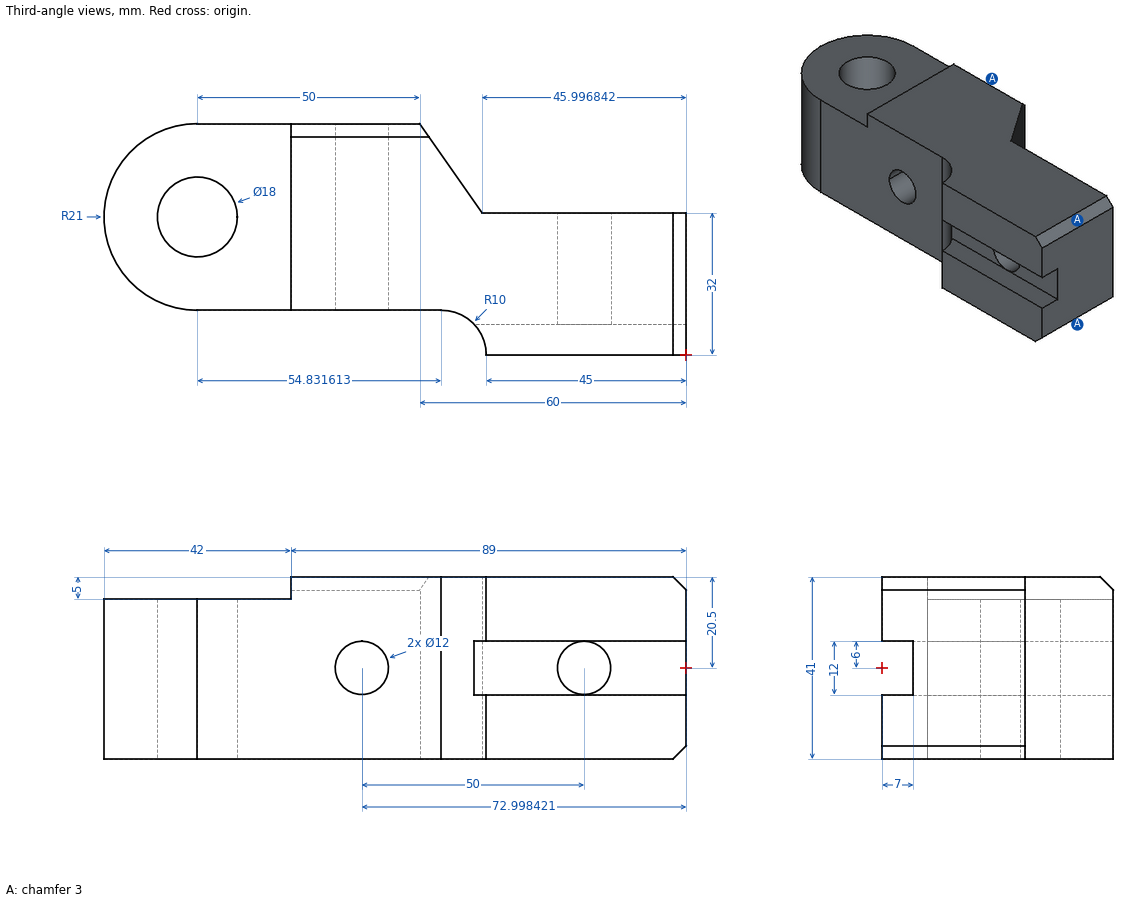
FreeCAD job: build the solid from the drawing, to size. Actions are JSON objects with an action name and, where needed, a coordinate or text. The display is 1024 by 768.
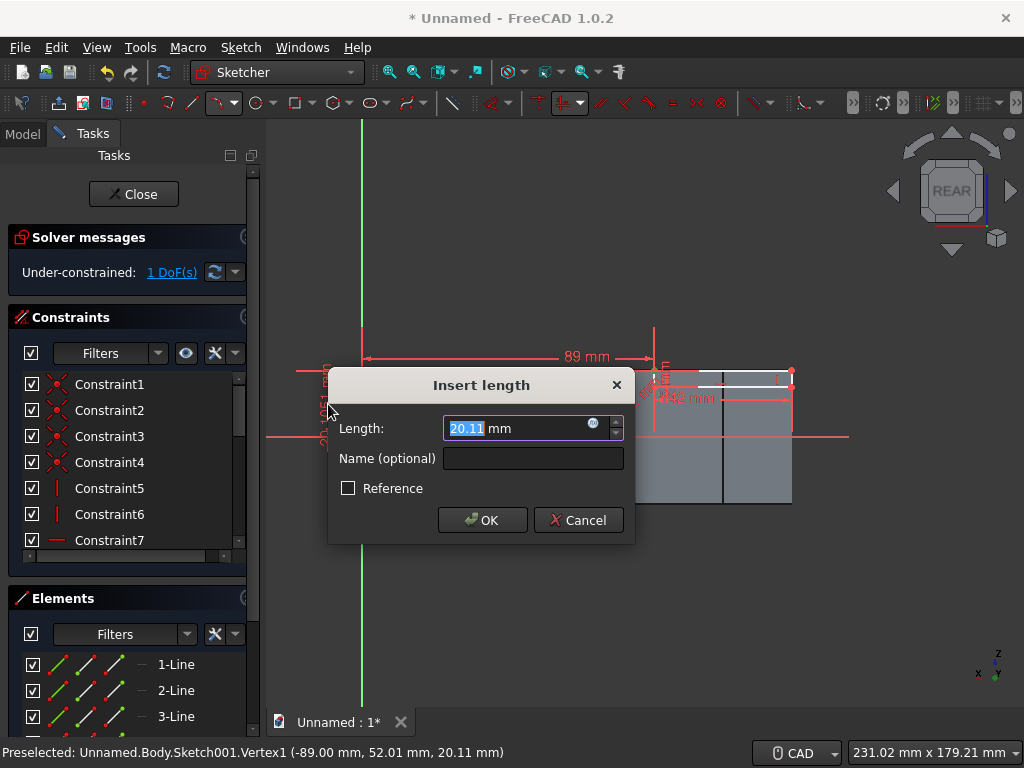
{"action": "type", "text": "20.5"}
{"action": "key", "text": "Return"}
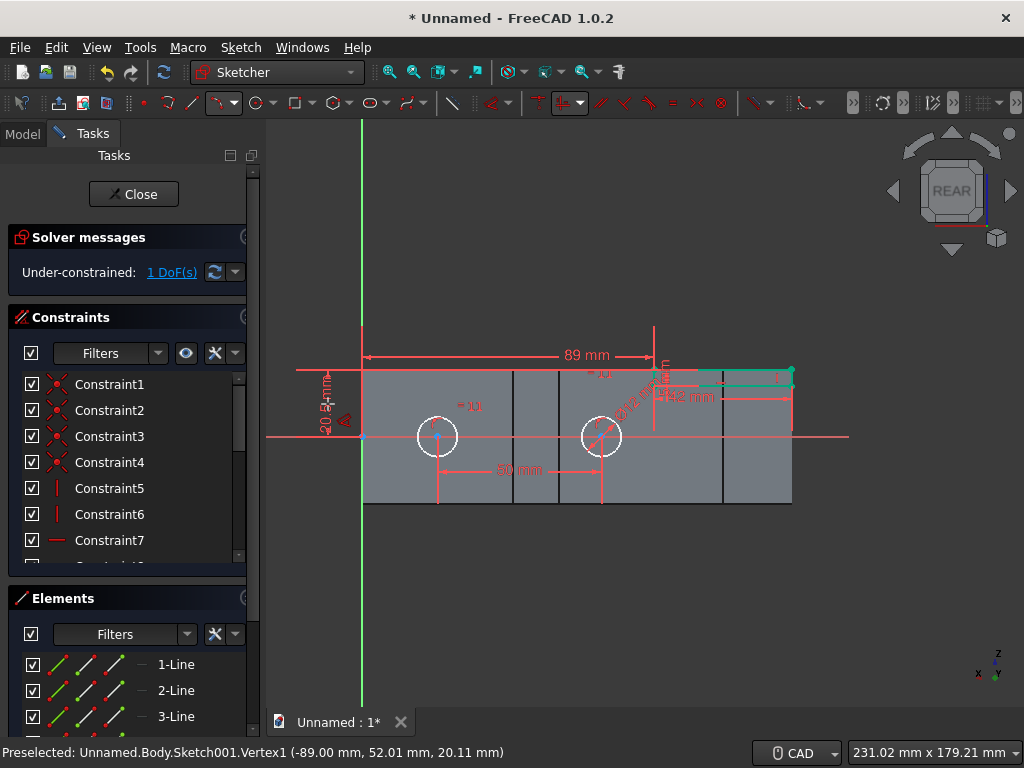
{"action": "left_click", "coordinate": [602, 437]}
{"action": "left_click", "coordinate": [427, 471]}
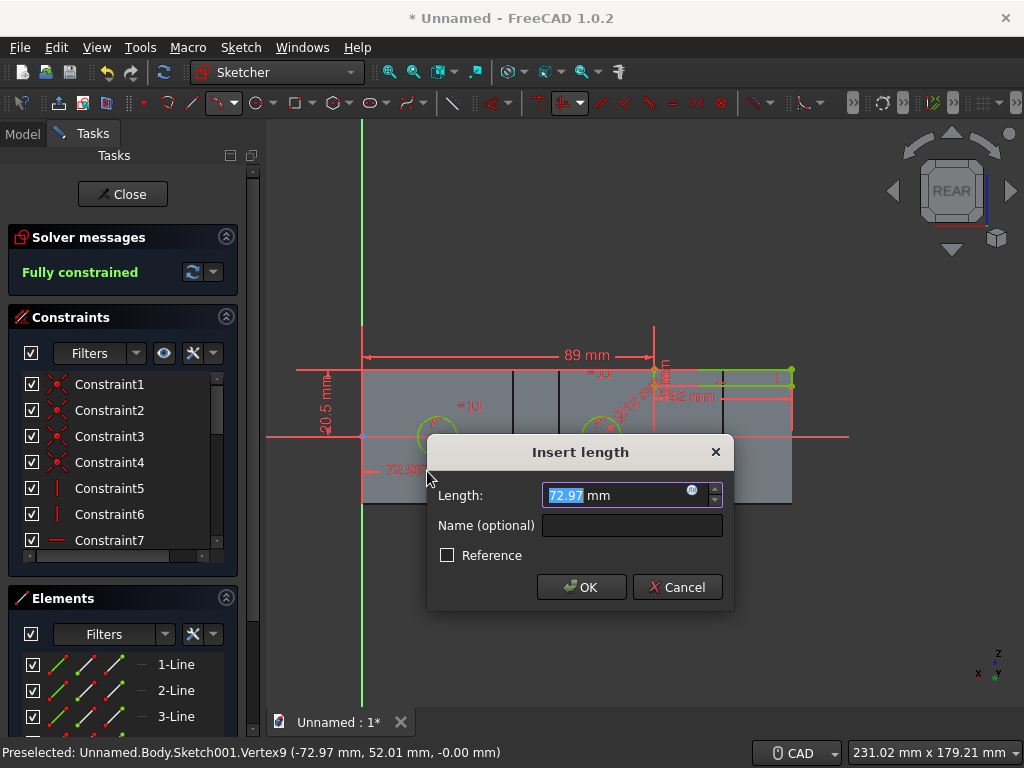
{"action": "type", "text": "72.998421"}
{"action": "key", "text": "Return"}
{"action": "key", "text": "Escape"}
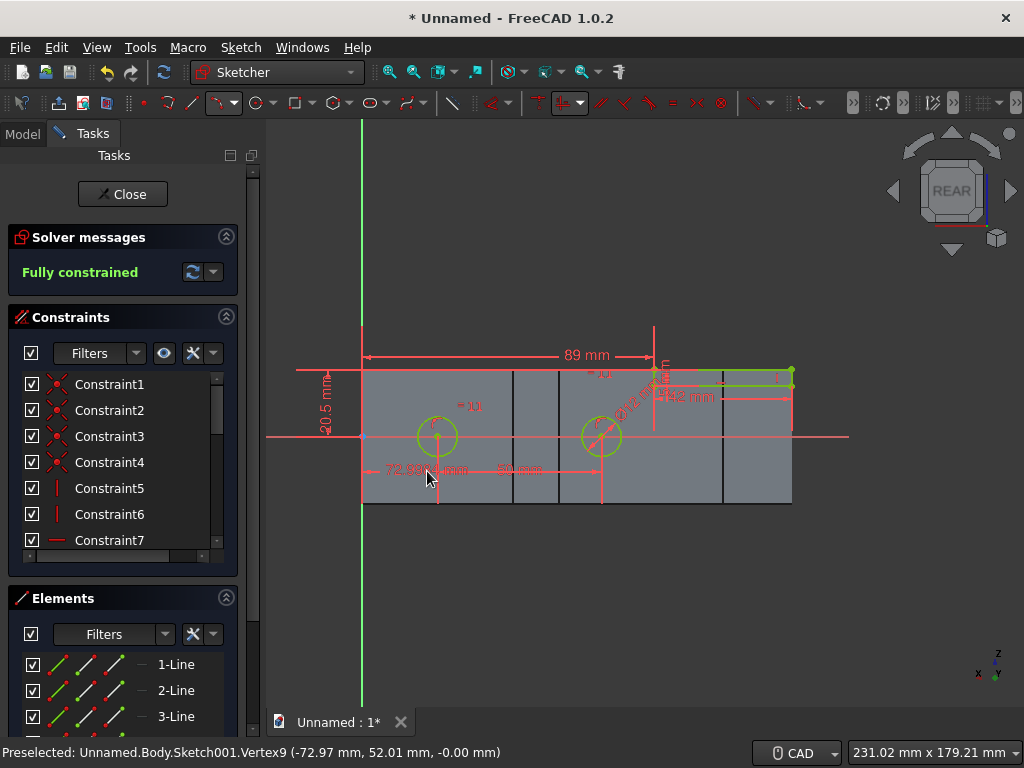
{"action": "left_click", "coordinate": [123, 194]}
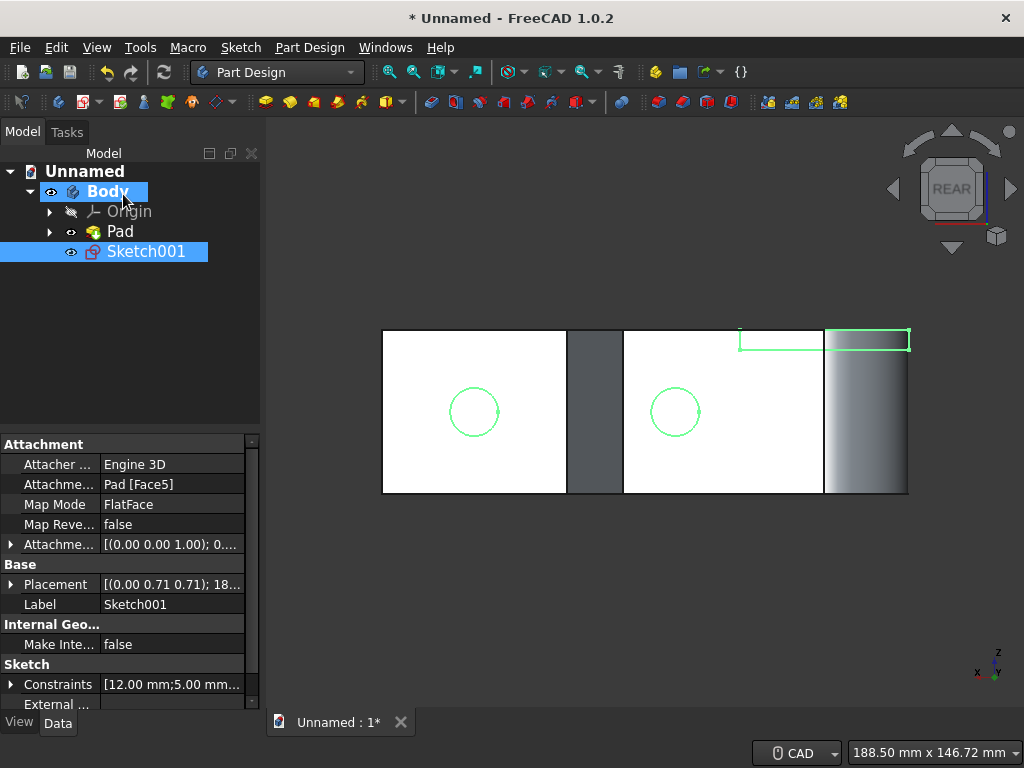
{"action": "left_click", "coordinate": [432, 102]}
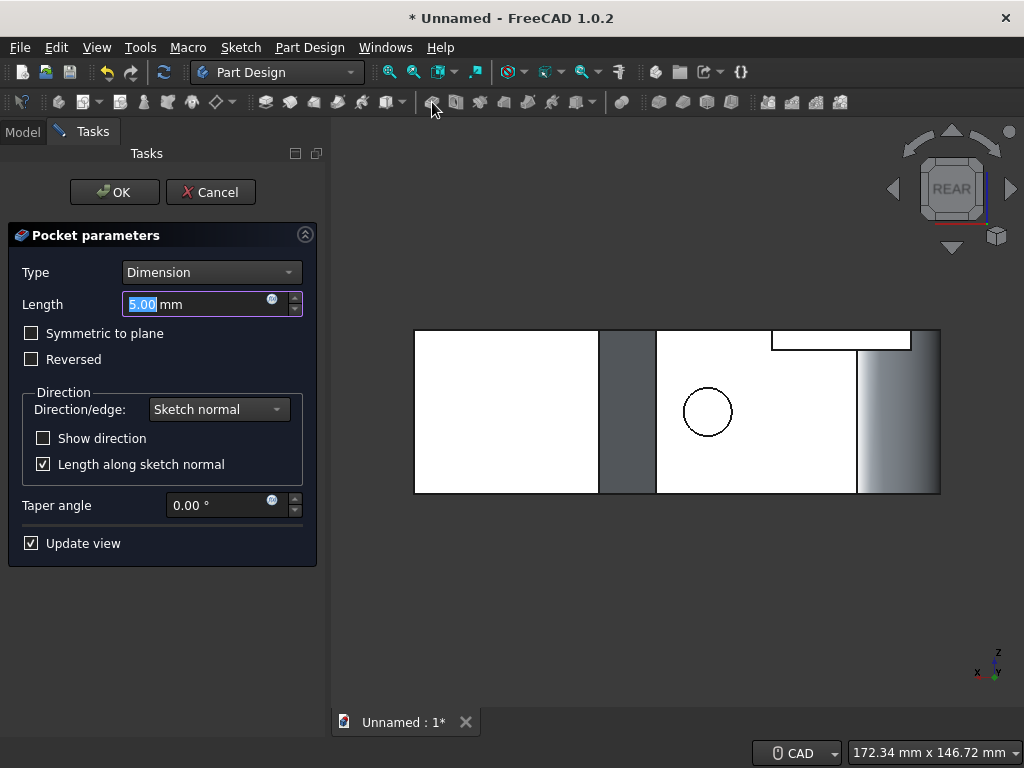
{"action": "left_click", "coordinate": [212, 272]}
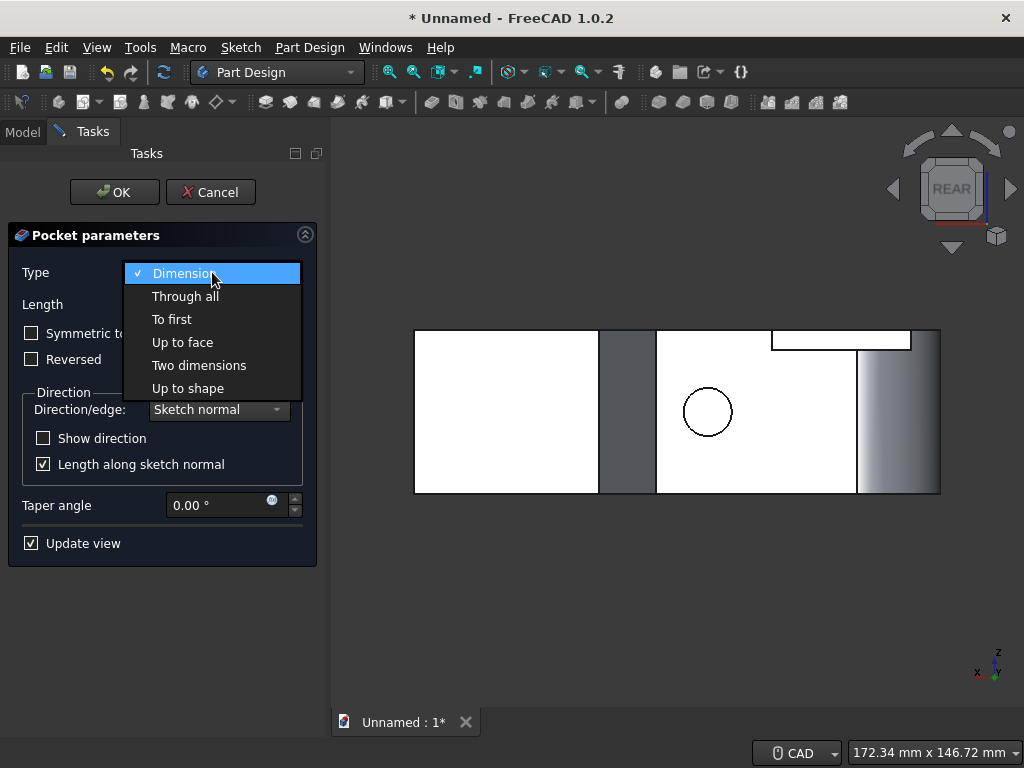
{"action": "left_click", "coordinate": [212, 296]}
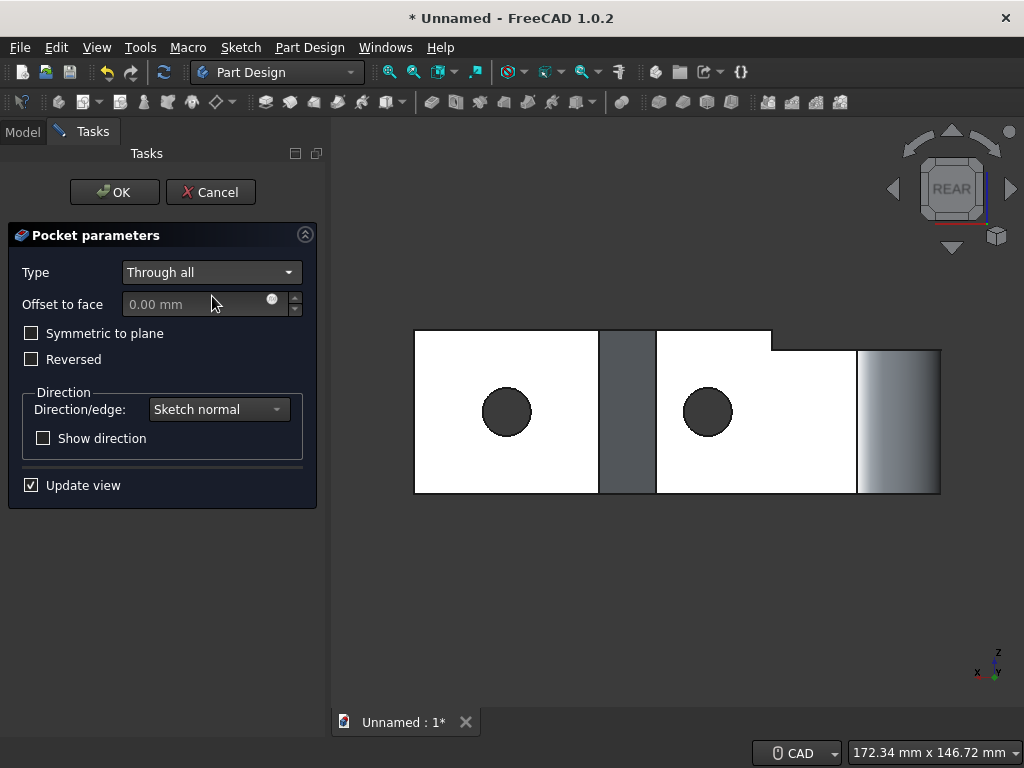
{"action": "left_click", "coordinate": [115, 192]}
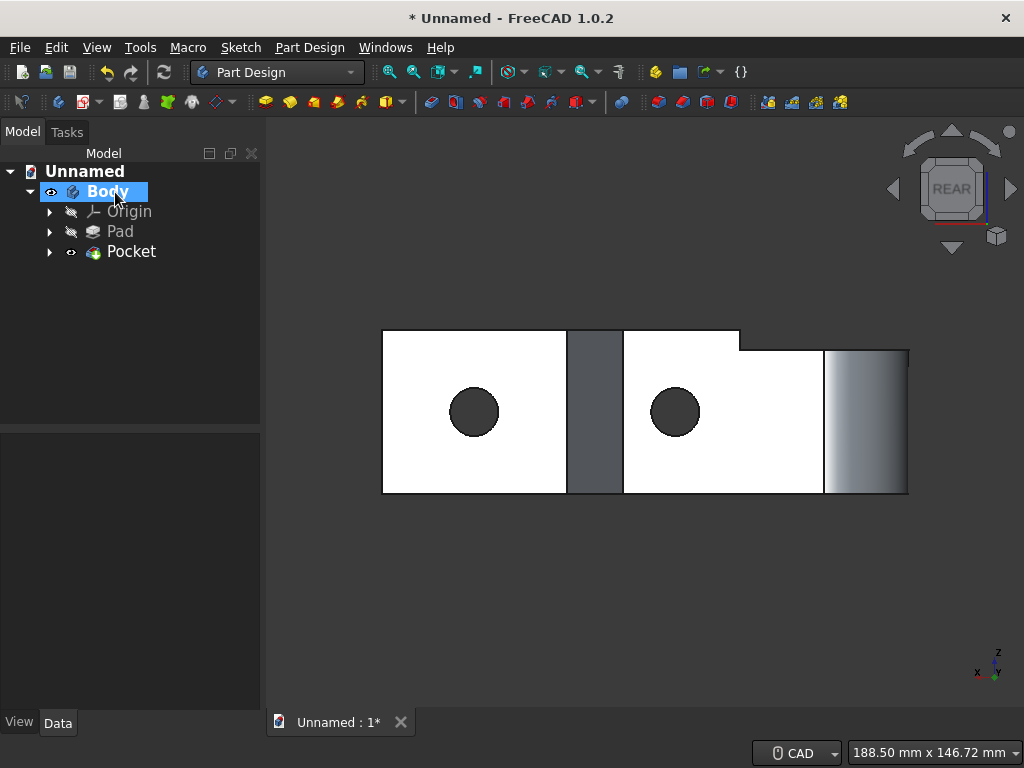
{"action": "left_click", "coordinate": [84, 102]}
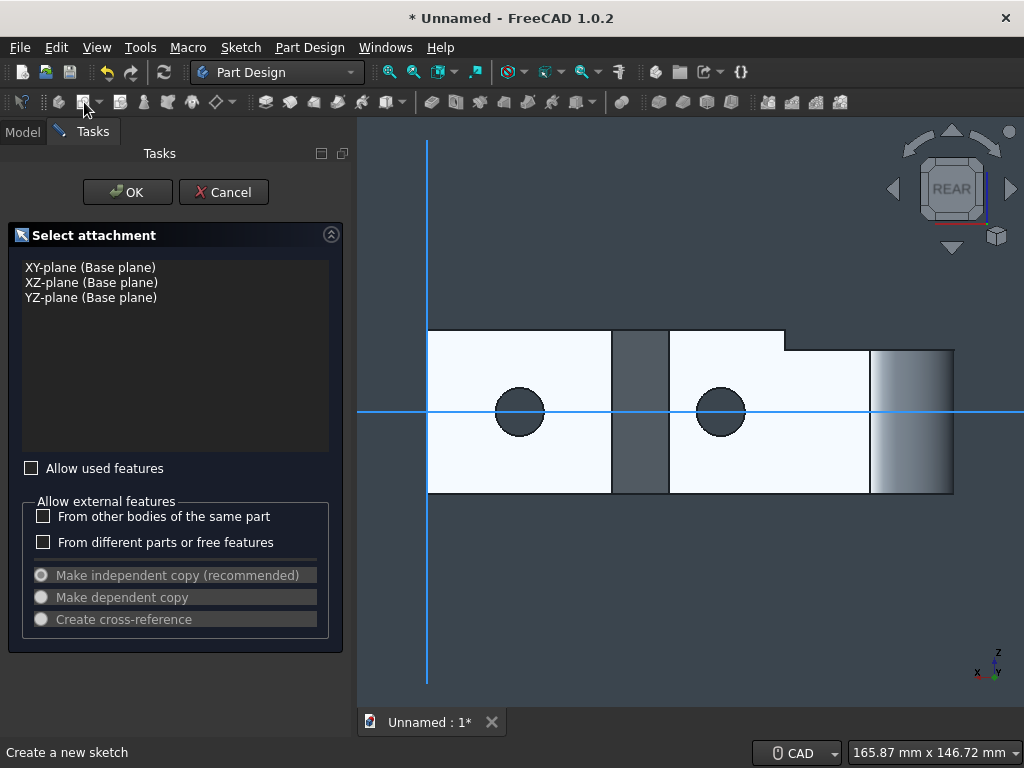
{"action": "left_click", "coordinate": [82, 298]}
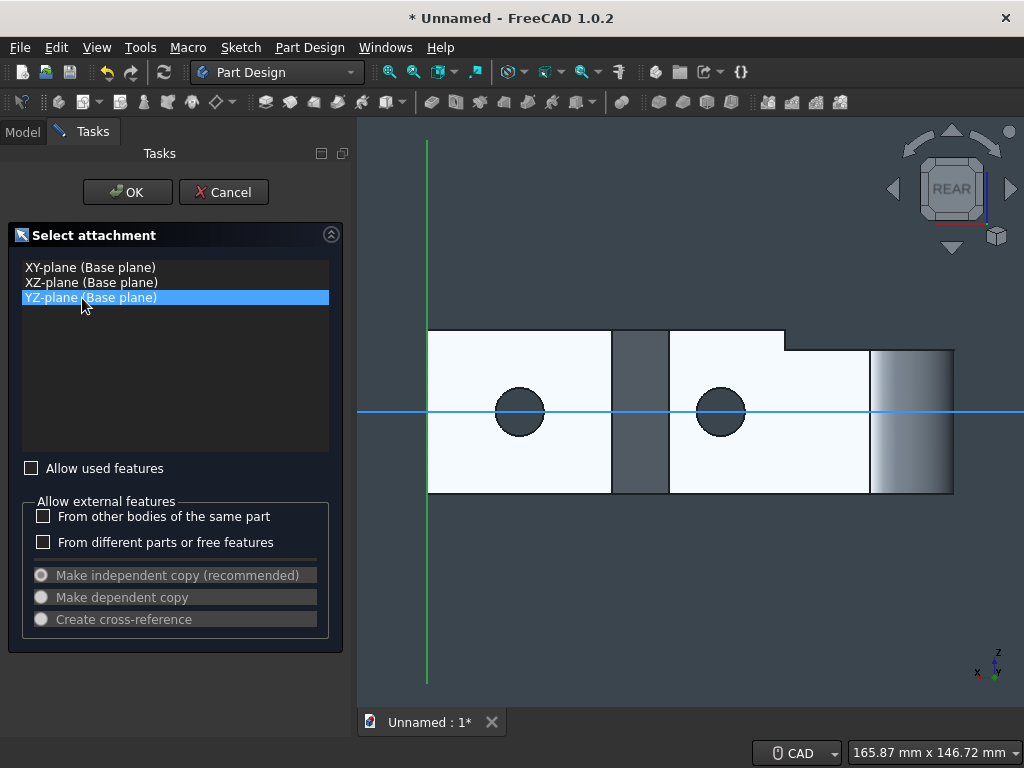
{"action": "left_click", "coordinate": [128, 192]}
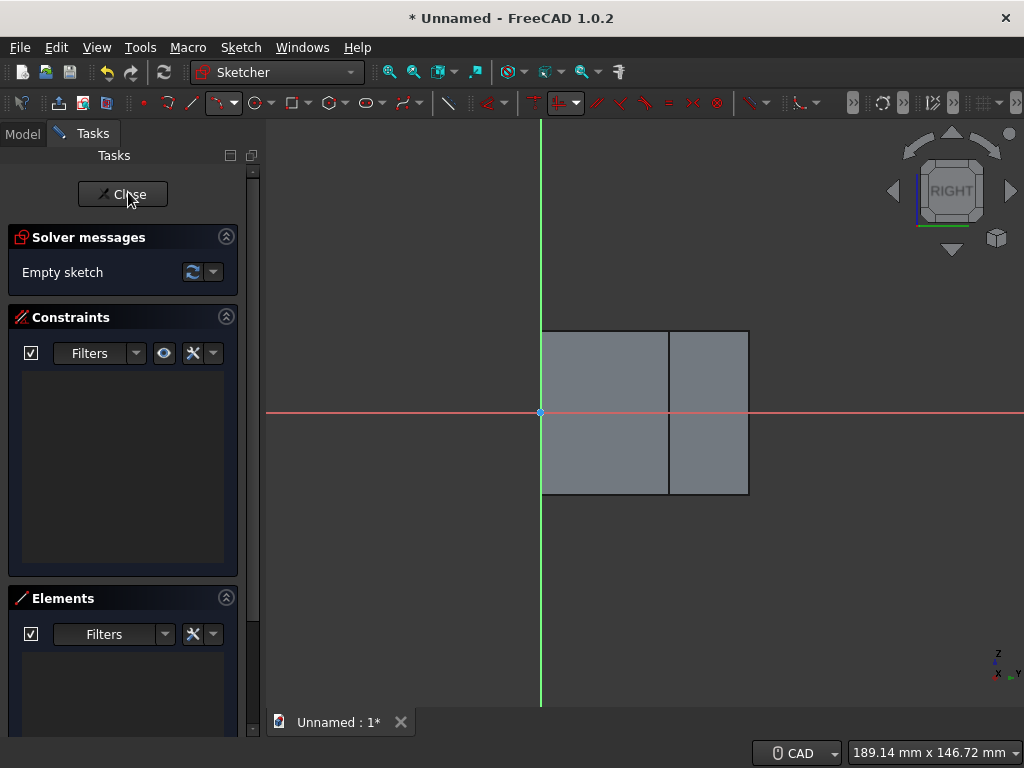
{"action": "scroll", "coordinate": [551, 413], "scroll_direction": "up", "scroll_amount": 10}